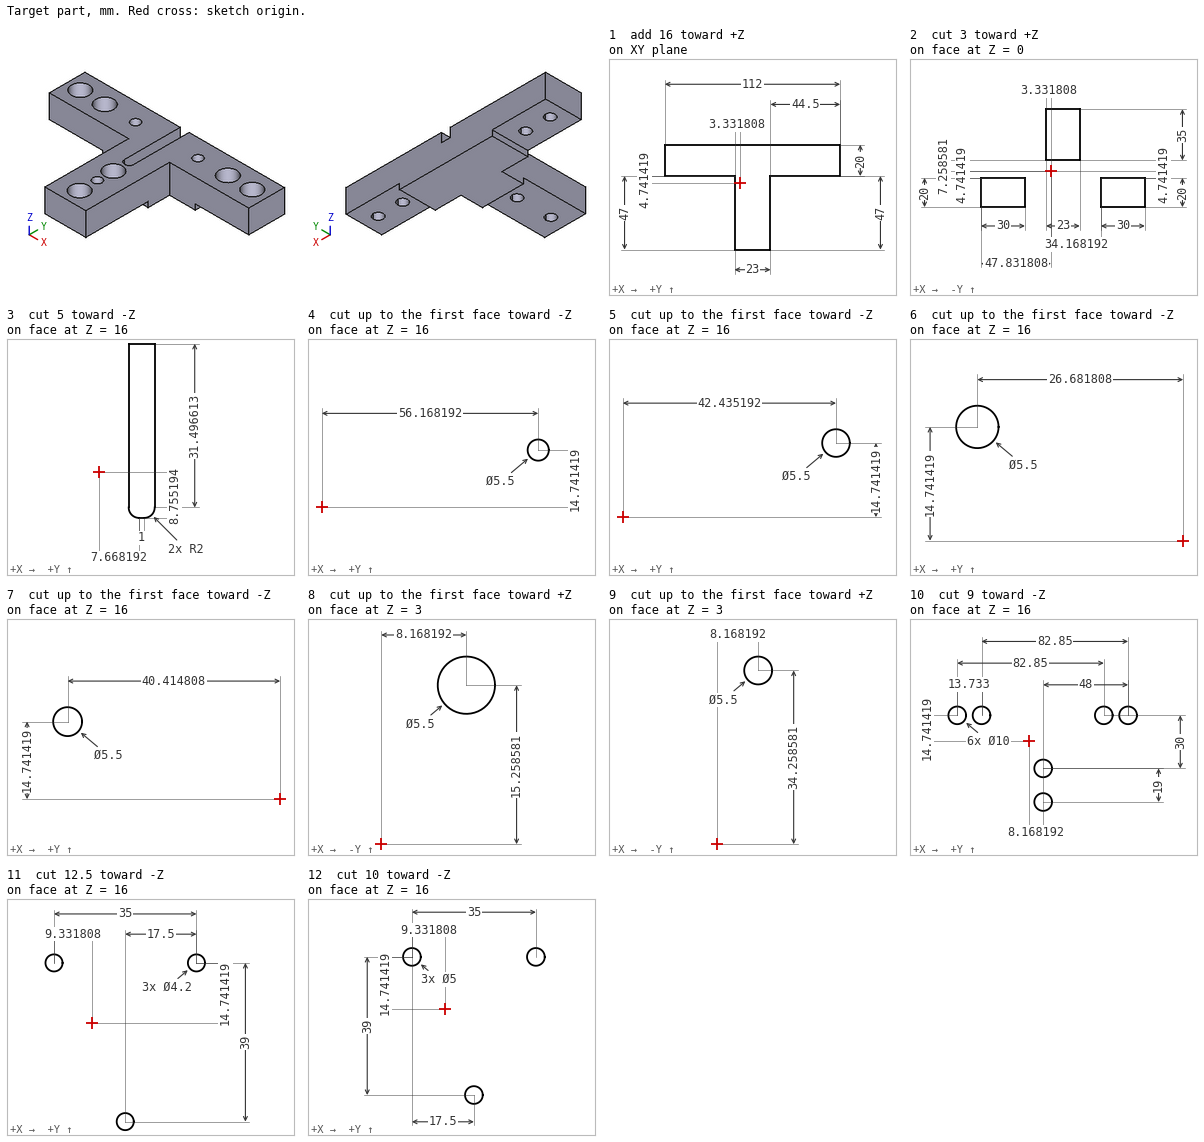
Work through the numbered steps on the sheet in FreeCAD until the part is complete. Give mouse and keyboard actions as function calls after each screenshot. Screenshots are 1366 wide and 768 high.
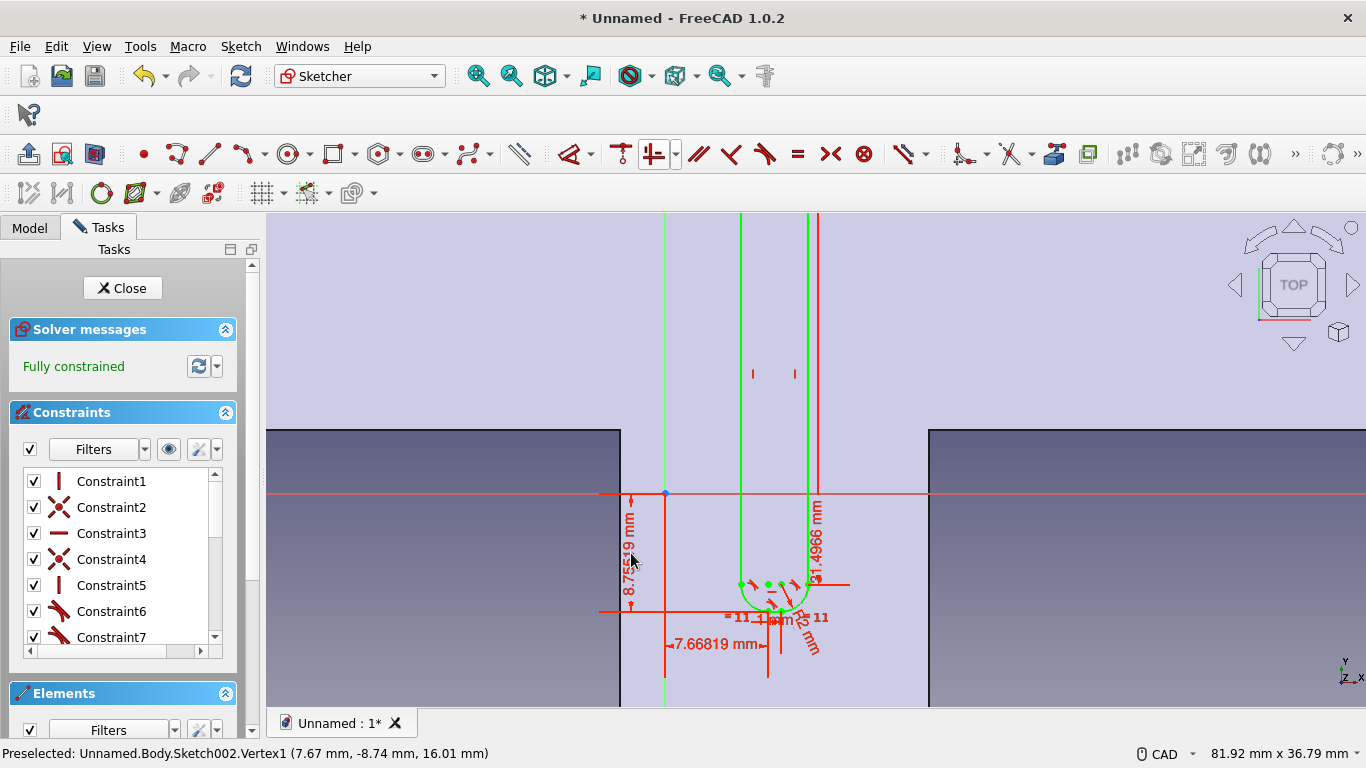
click(123, 288)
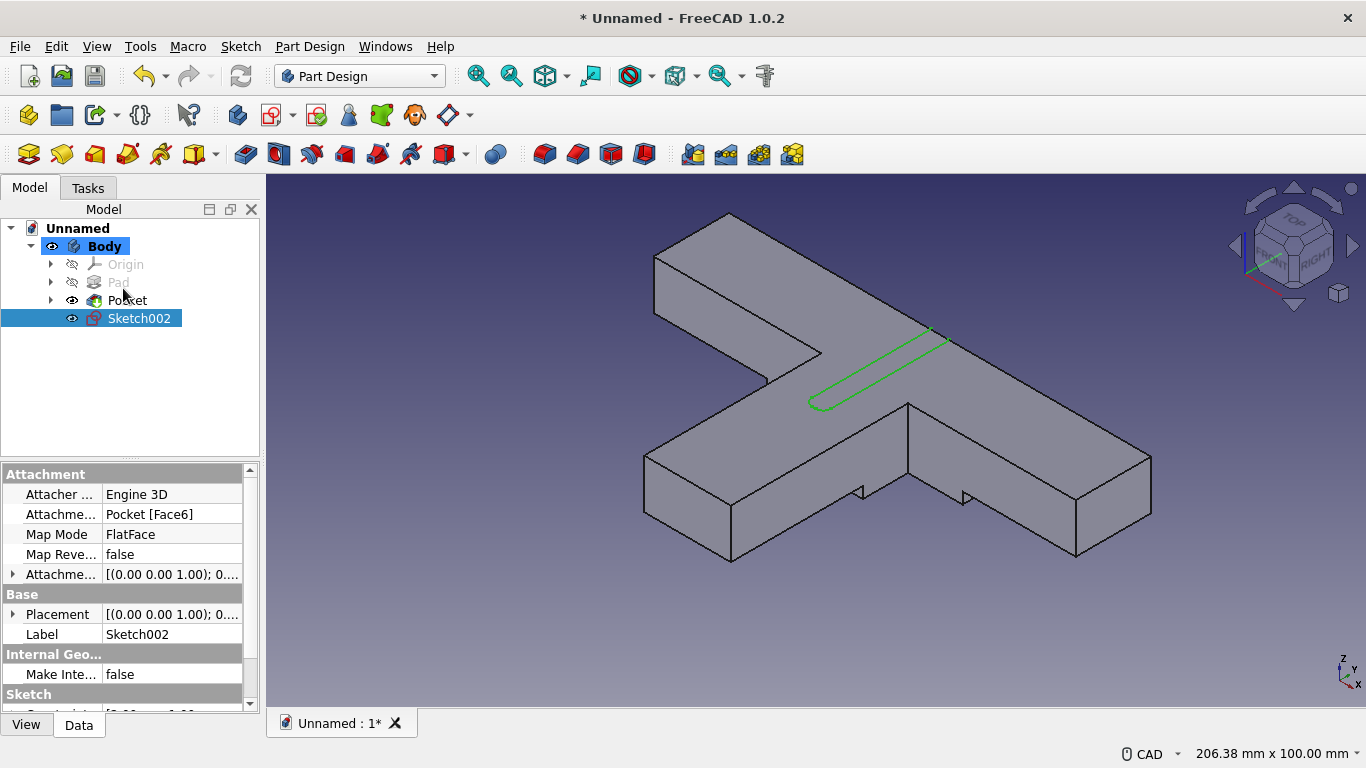
click(246, 154)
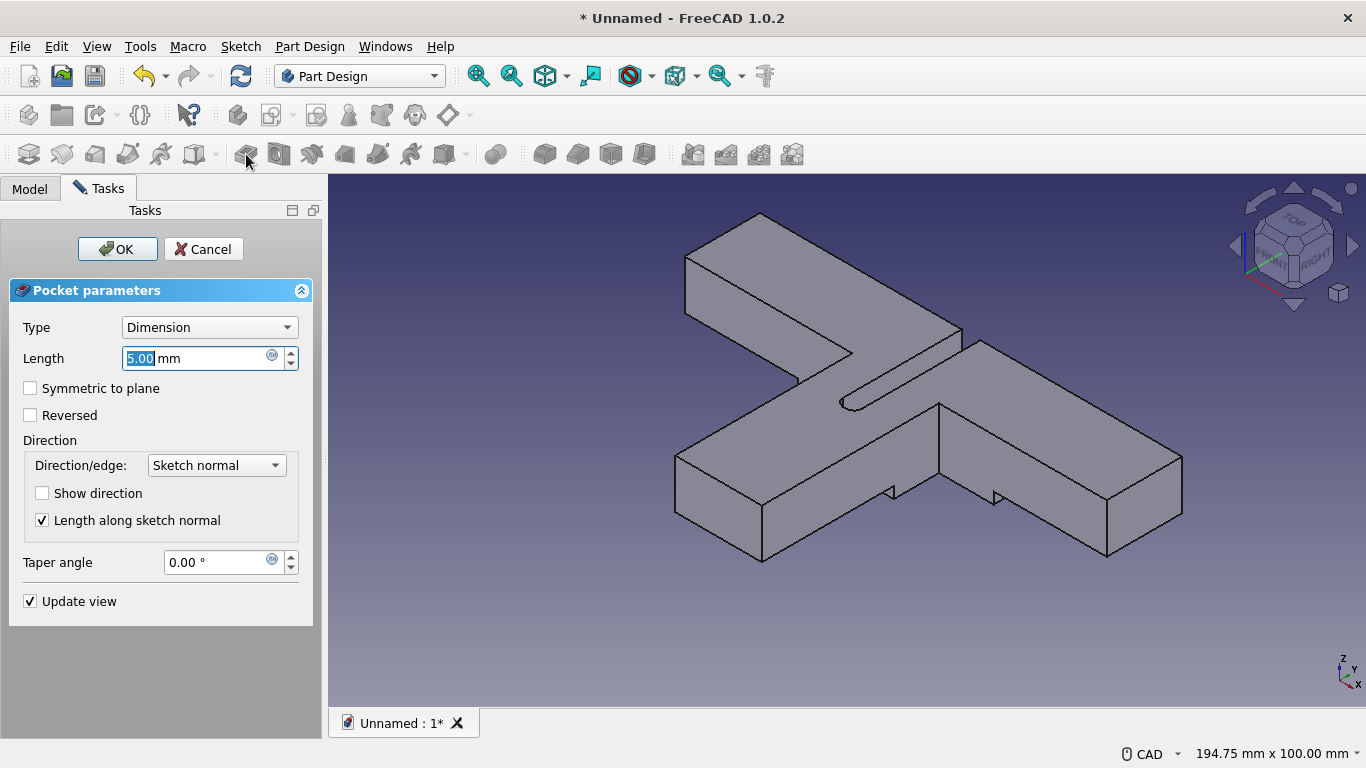
text(5)
key(Tab)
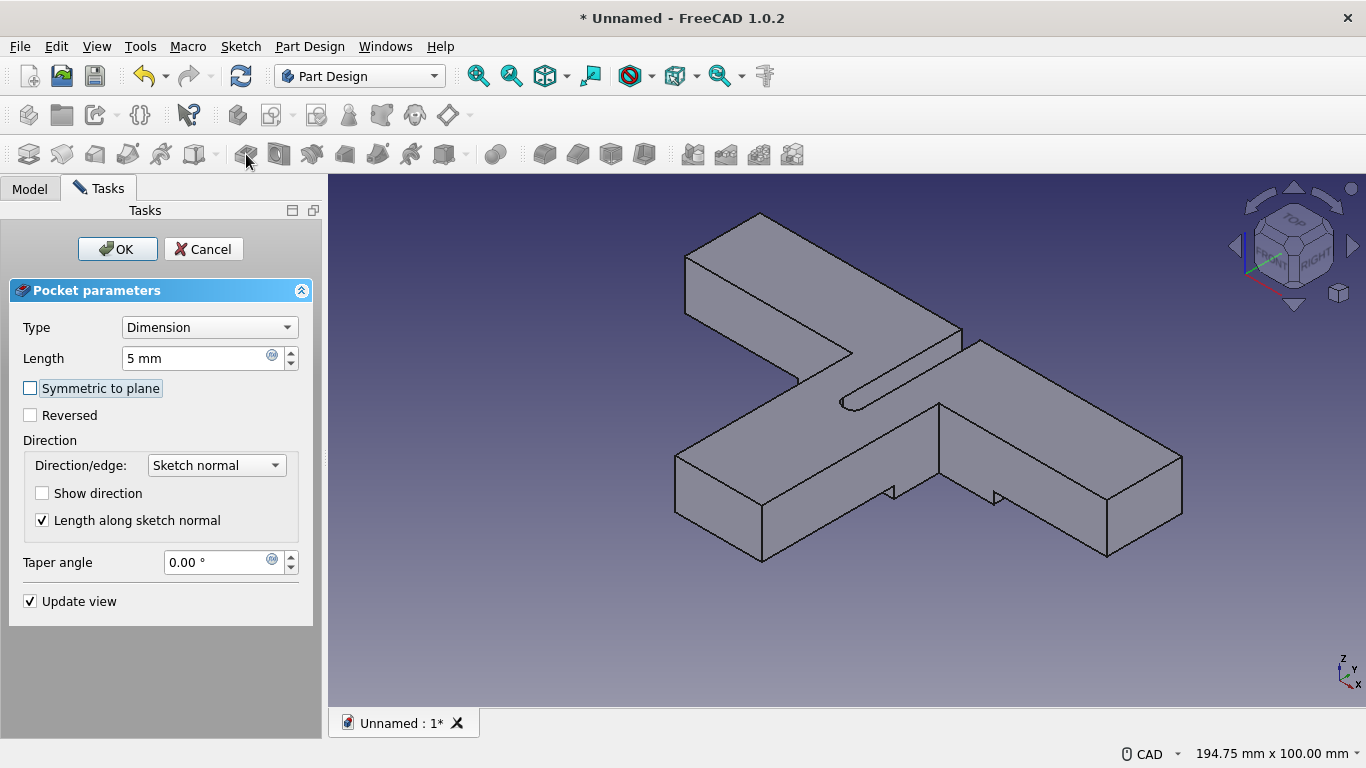
click(118, 249)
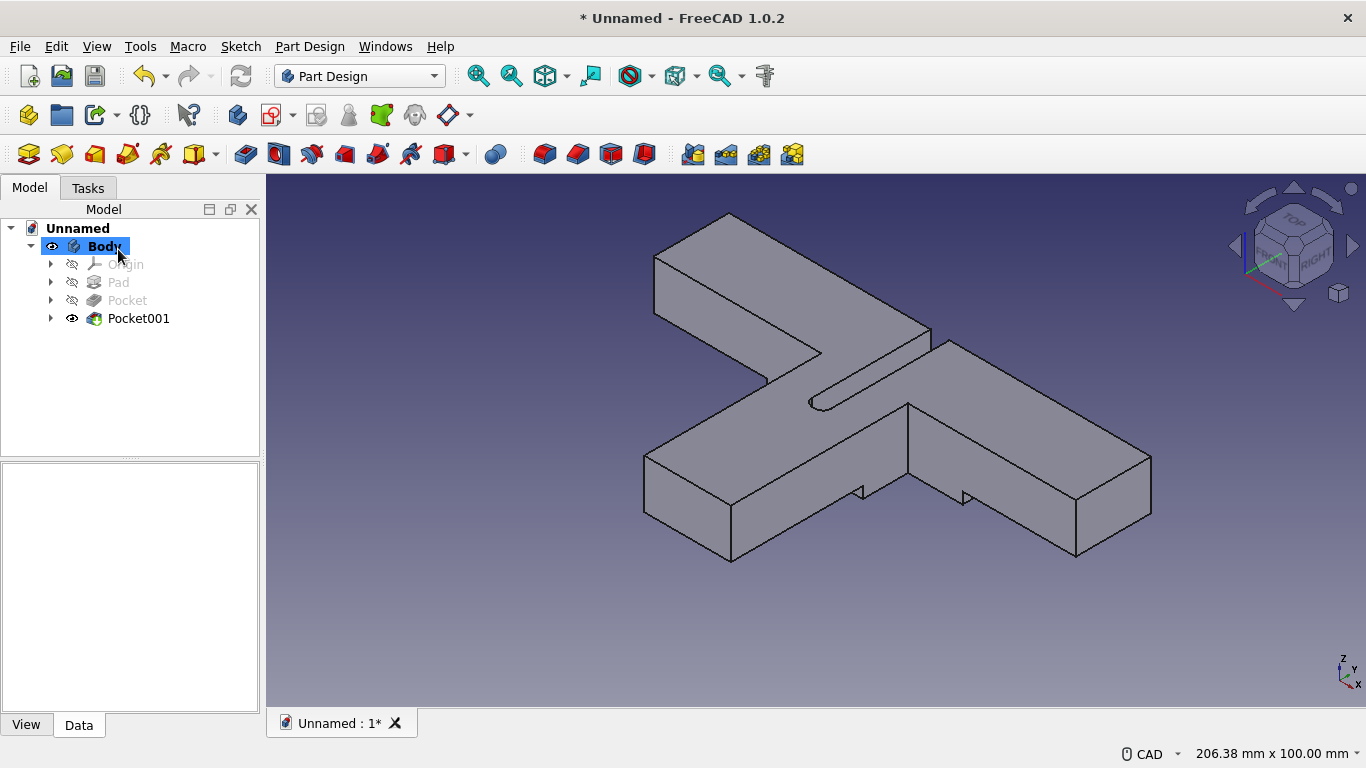
click(742, 448)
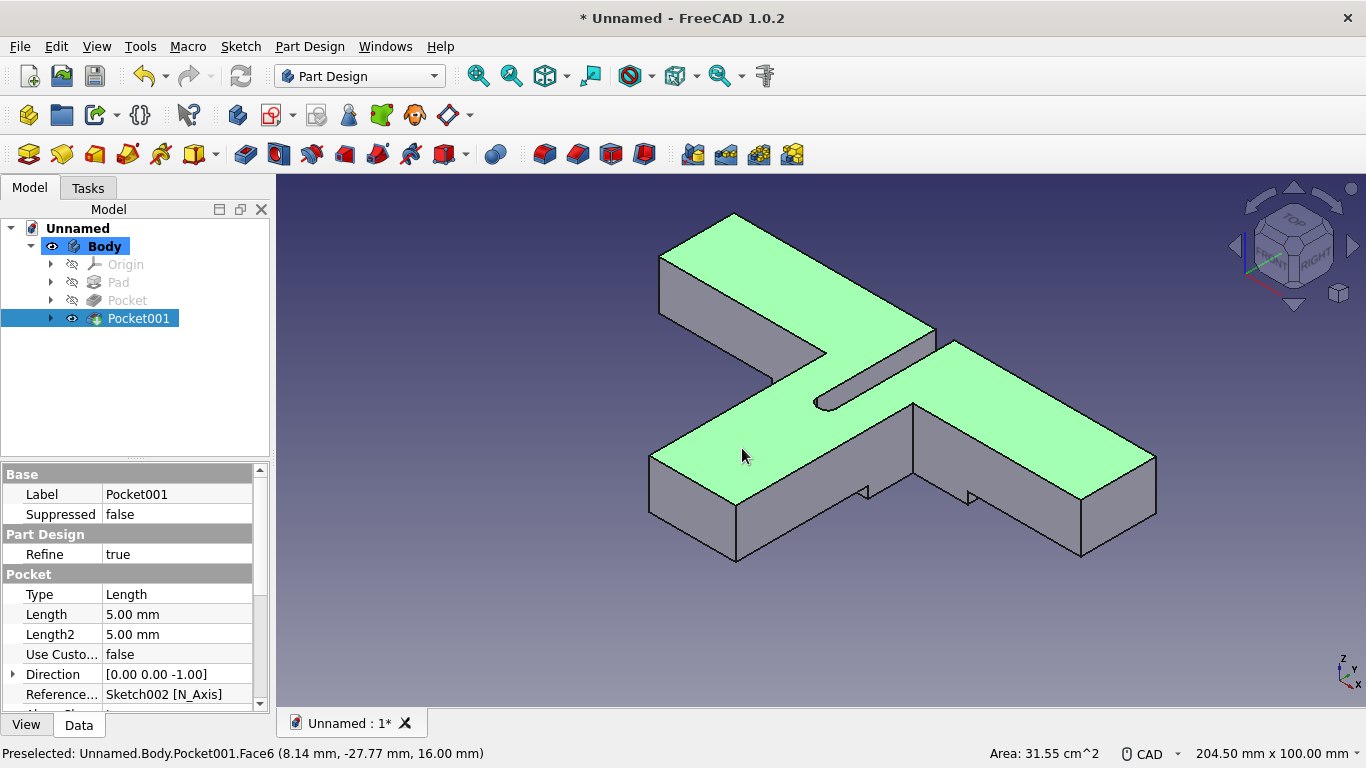
click(270, 116)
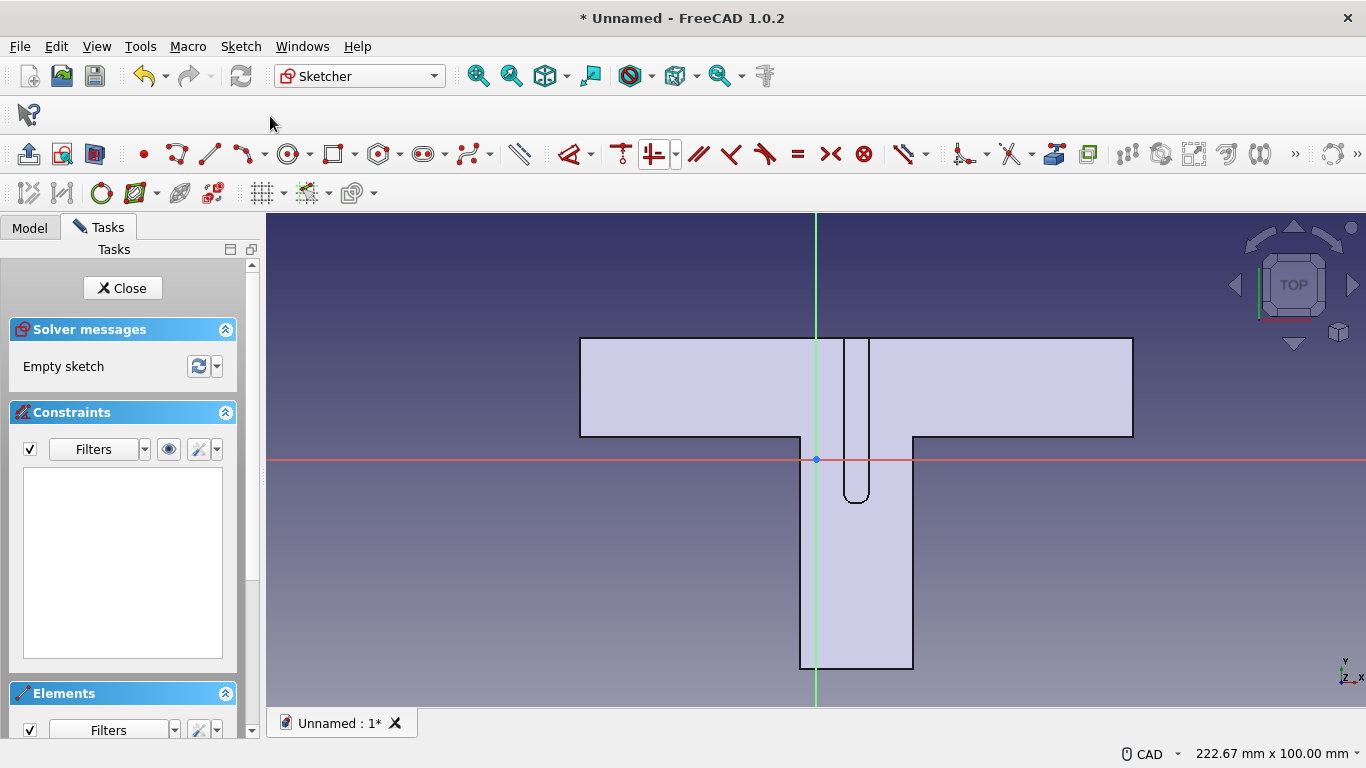
scroll(1128, 380, up, 12)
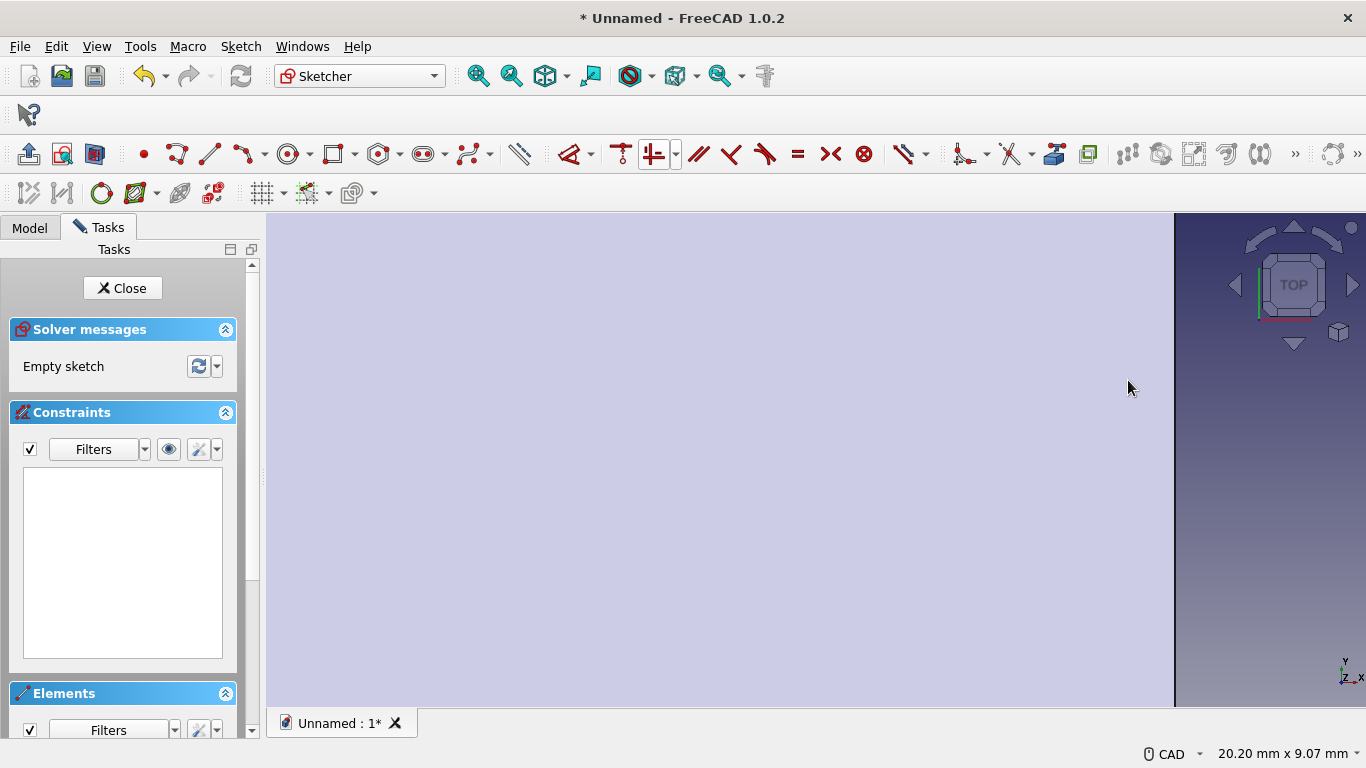
key(g)
key(c)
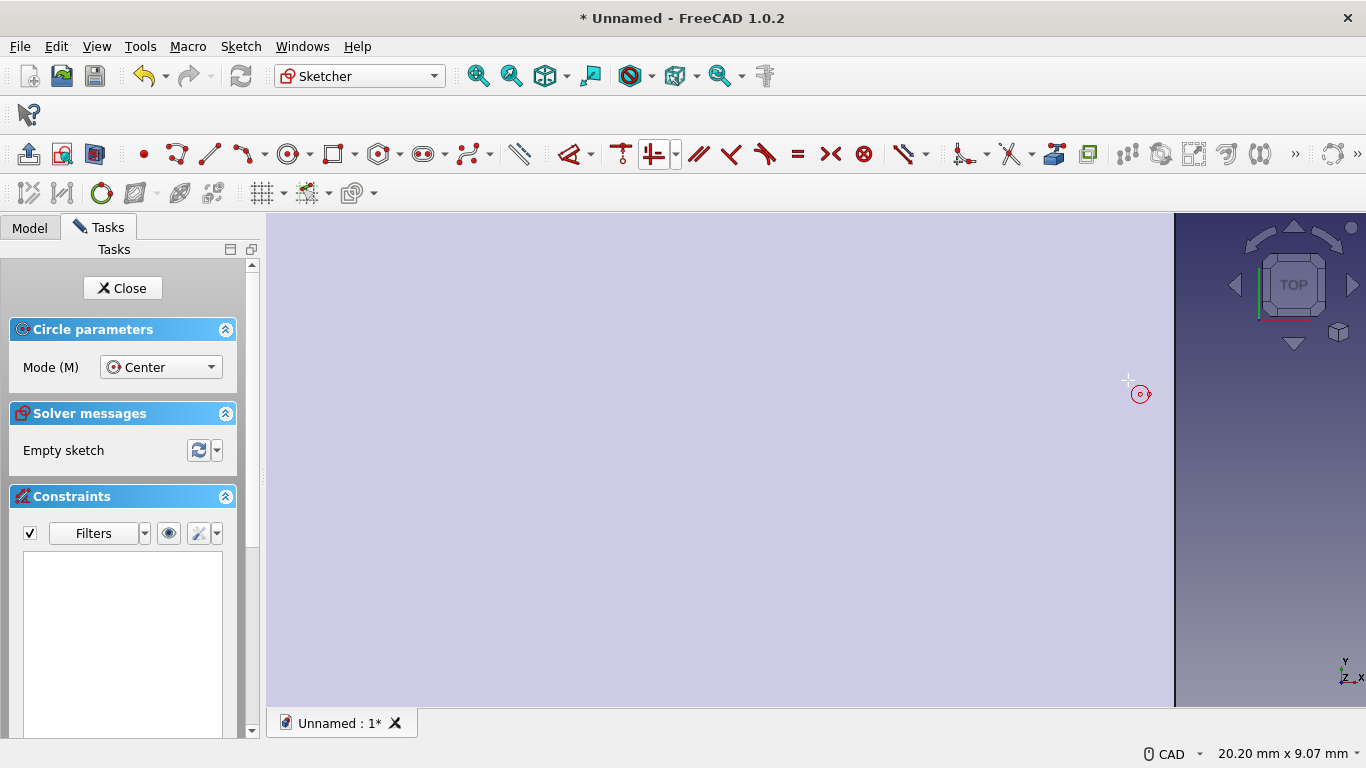
click(740, 456)
move(845, 350)